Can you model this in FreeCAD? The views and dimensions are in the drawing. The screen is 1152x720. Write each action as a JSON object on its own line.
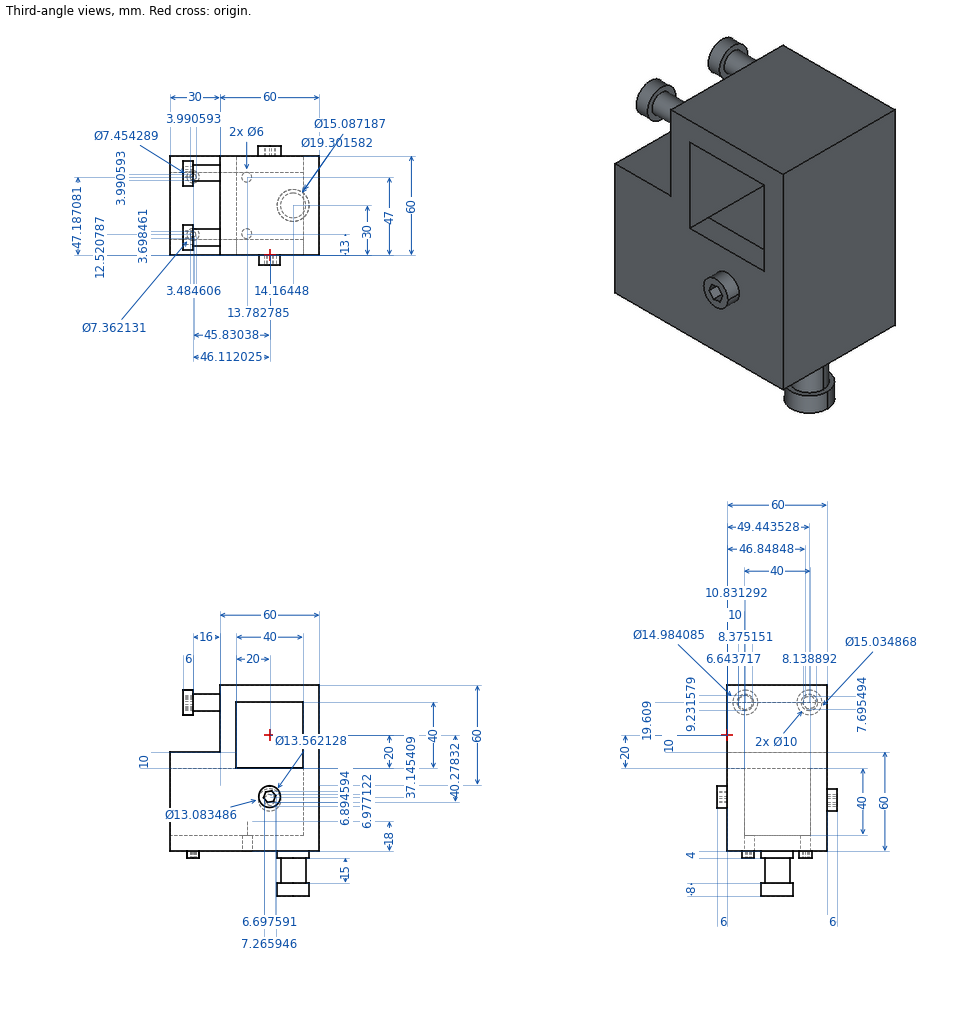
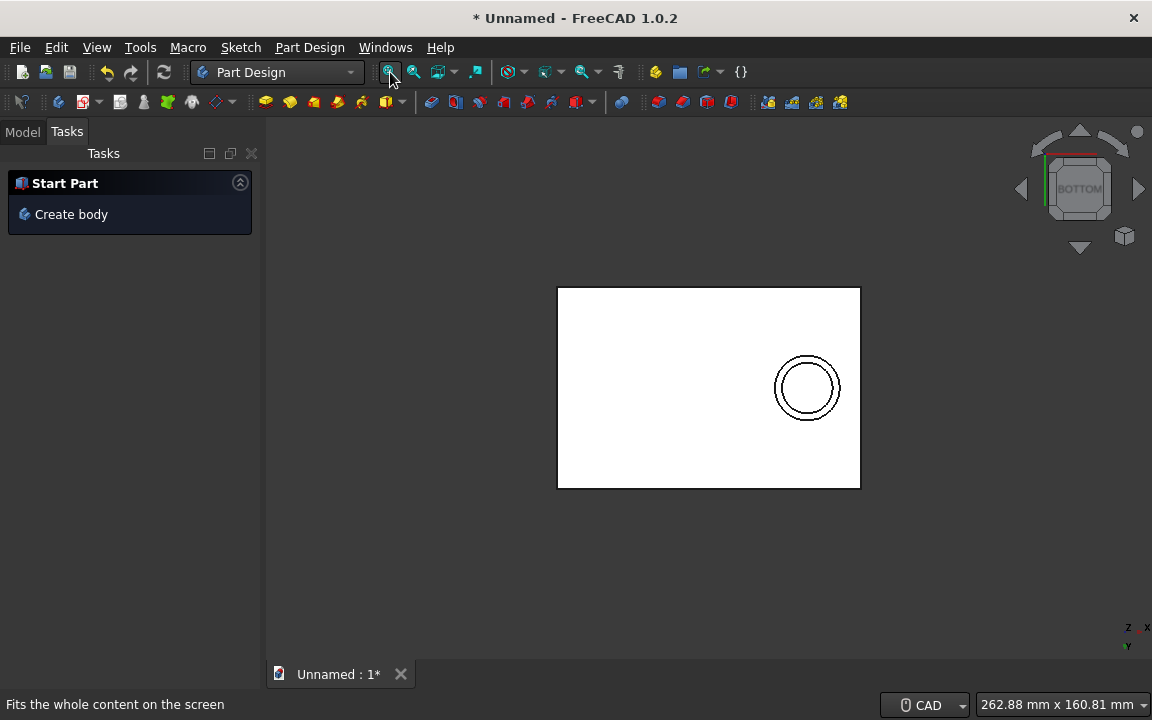
{"action": "left_click", "coordinate": [807, 387]}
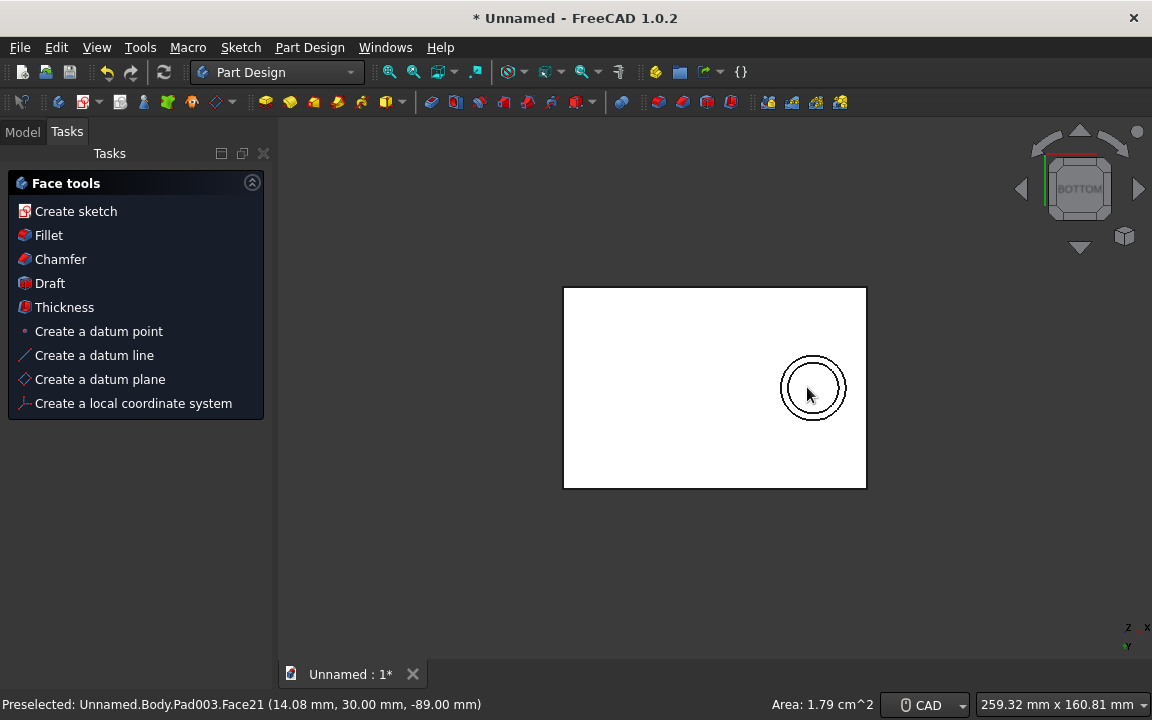
{"action": "left_click", "coordinate": [84, 102]}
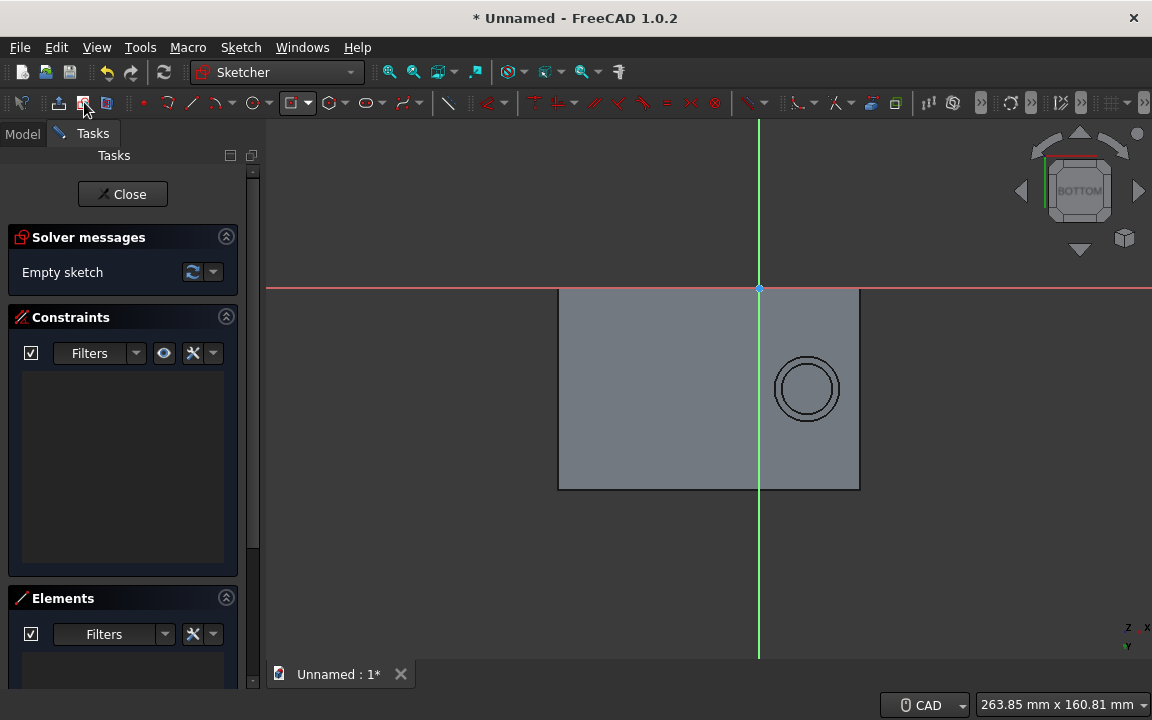
{"action": "scroll", "coordinate": [892, 335], "scroll_direction": "up", "scroll_amount": 5}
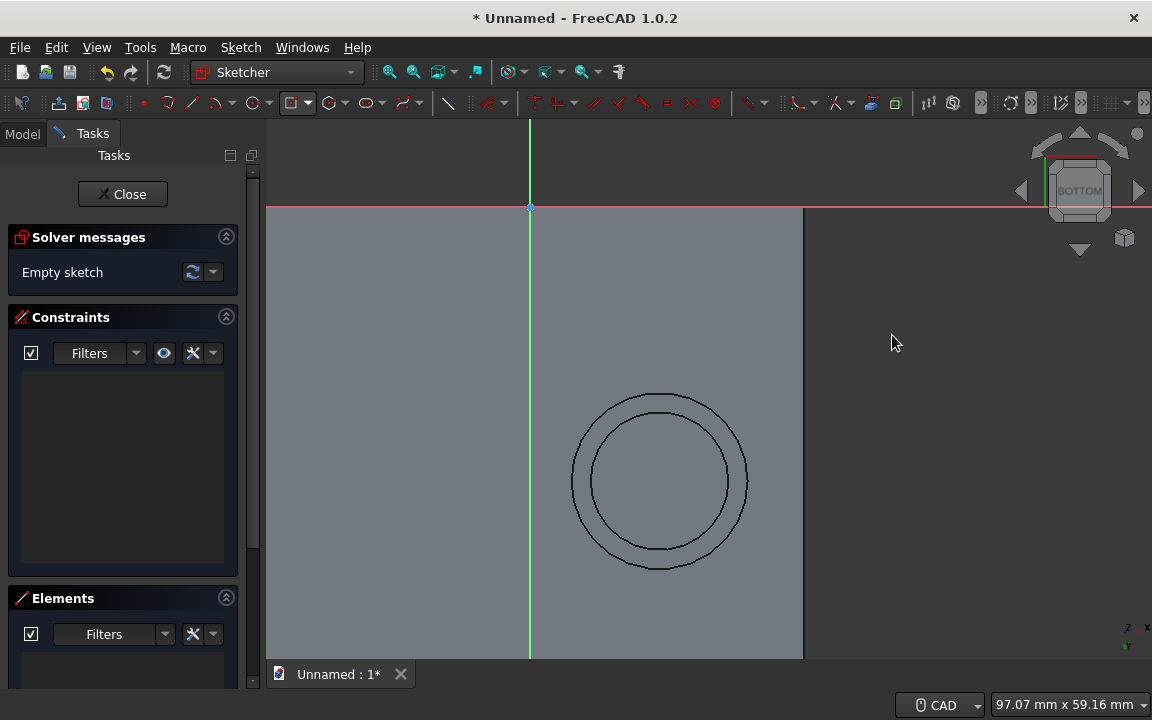
{"action": "left_click", "coordinate": [254, 104]}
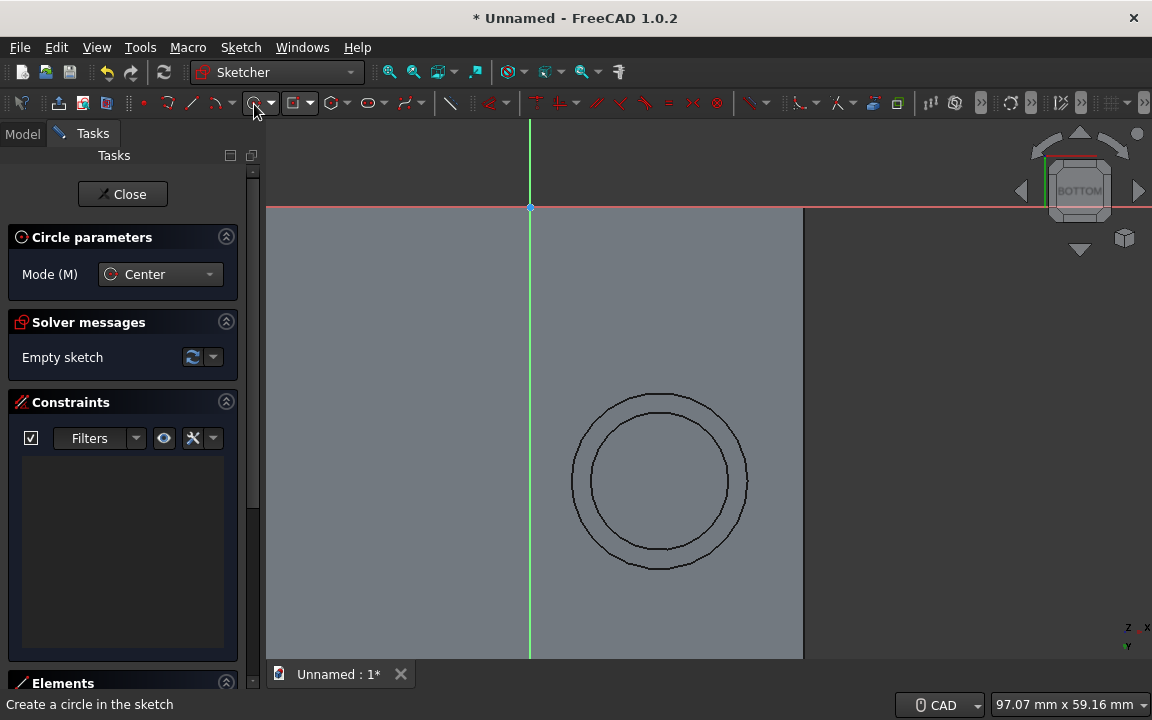
{"action": "left_click", "coordinate": [660, 481]}
{"action": "left_click", "coordinate": [722, 419]}
{"action": "key", "text": "Escape"}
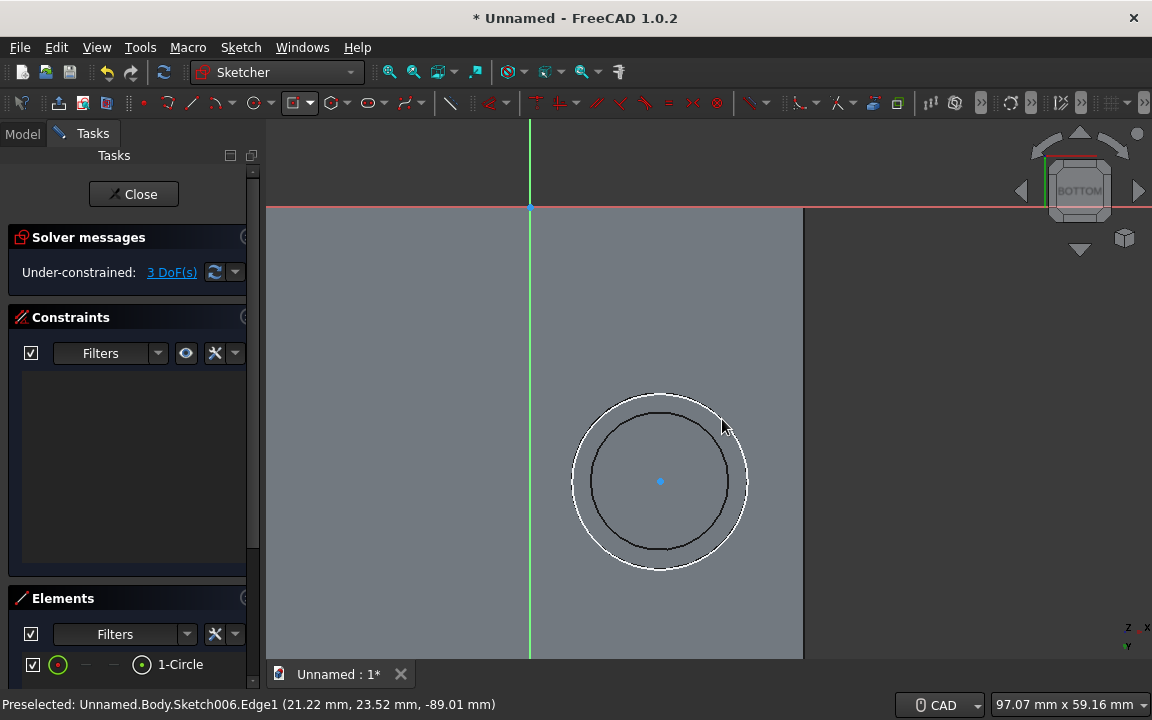
{"action": "left_click", "coordinate": [490, 104]}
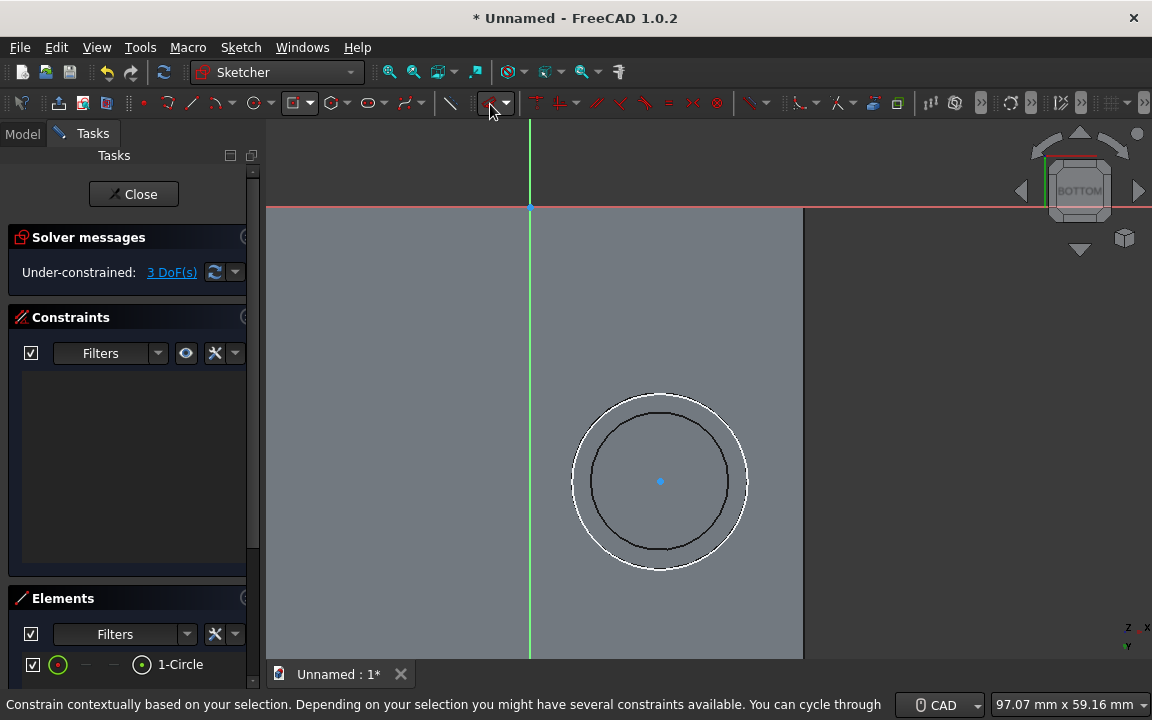
{"action": "left_click", "coordinate": [722, 420]}
{"action": "left_click", "coordinate": [745, 397]}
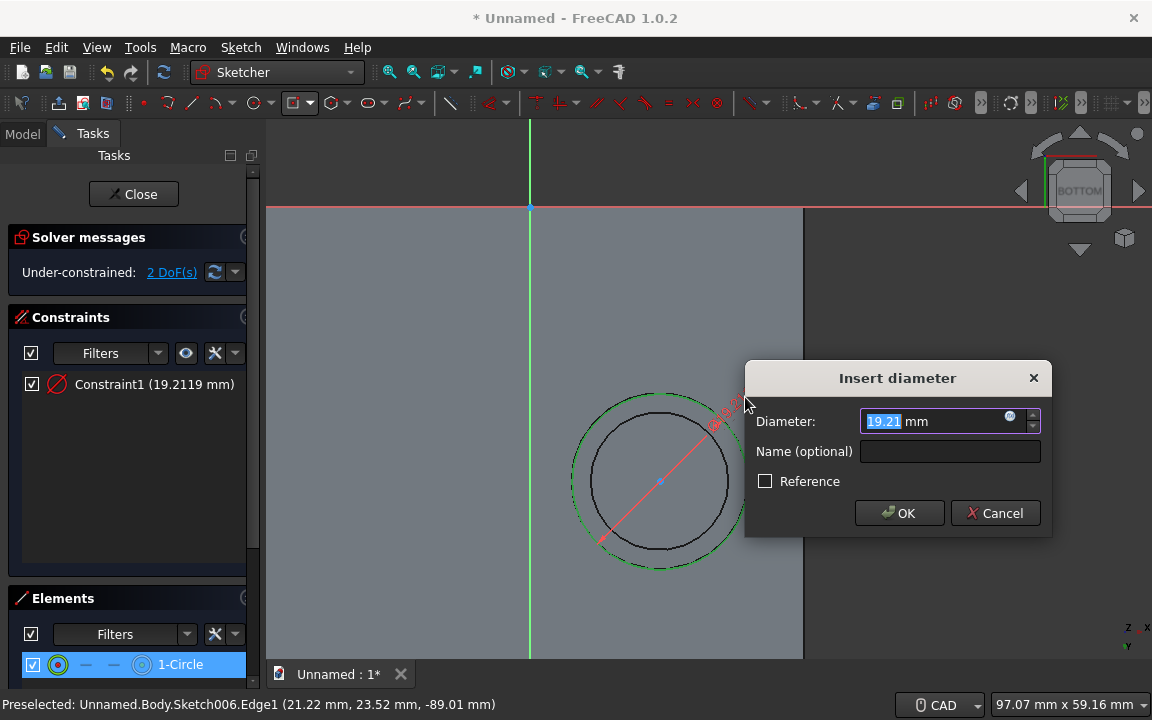
{"action": "type", "text": "19.301582"}
{"action": "key", "text": "Return"}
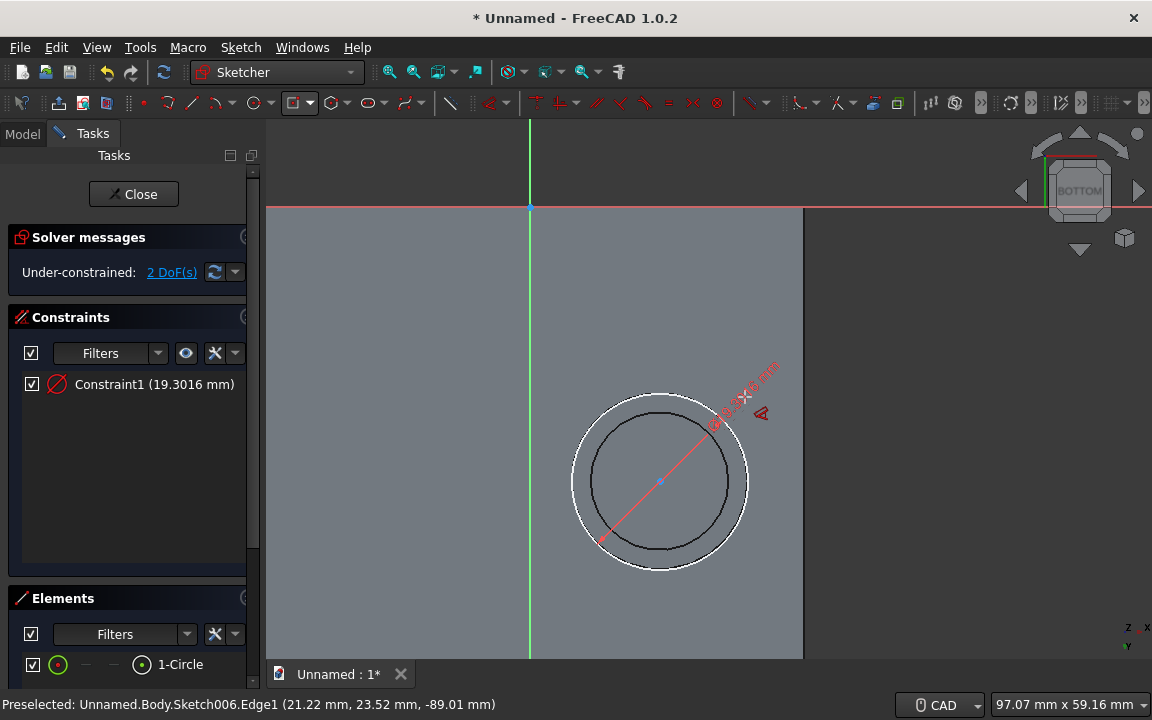
{"action": "left_click", "coordinate": [660, 482]}
{"action": "left_click", "coordinate": [496, 345]}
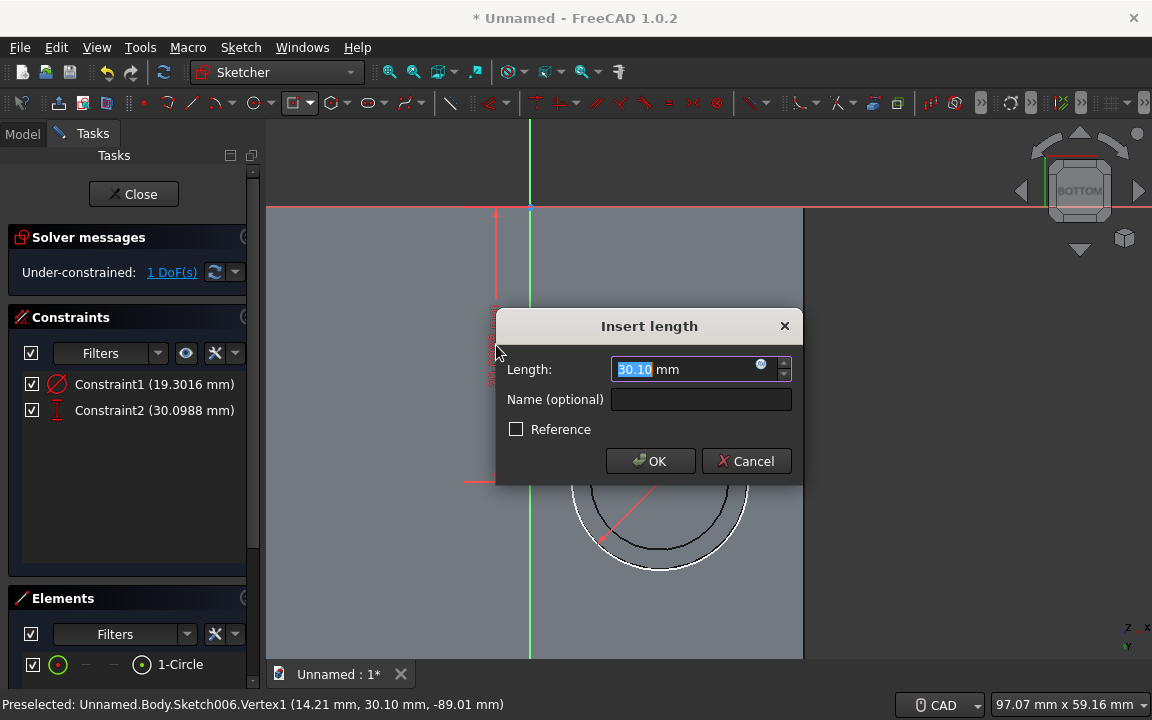
{"action": "type", "text": "30"}
{"action": "key", "text": "Return"}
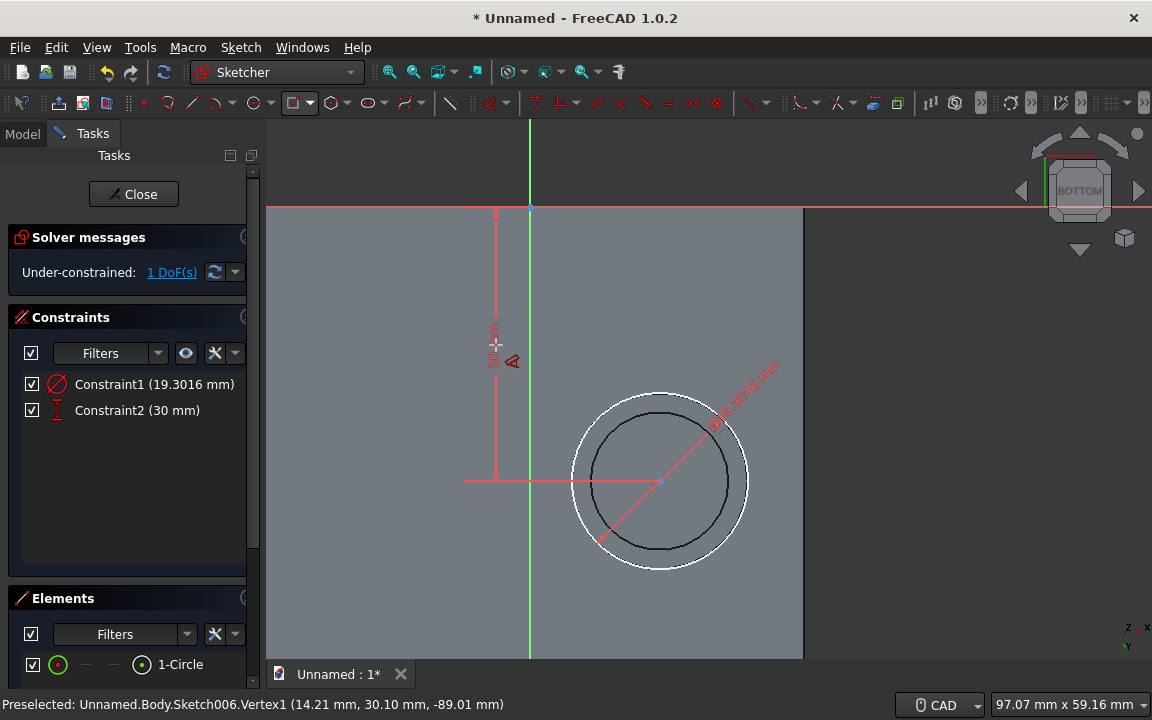
{"action": "left_click", "coordinate": [660, 481]}
{"action": "left_click", "coordinate": [595, 173]}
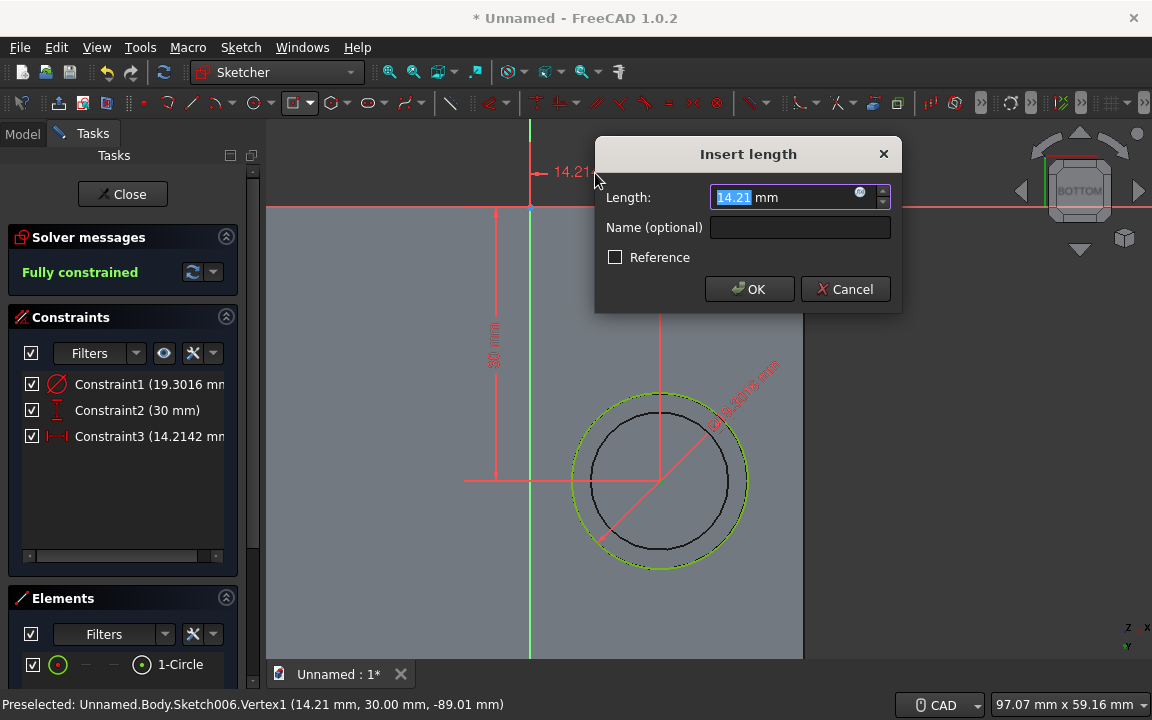
{"action": "type", "text": "14.16448"}
{"action": "key", "text": "Return"}
{"action": "key", "text": "Escape"}